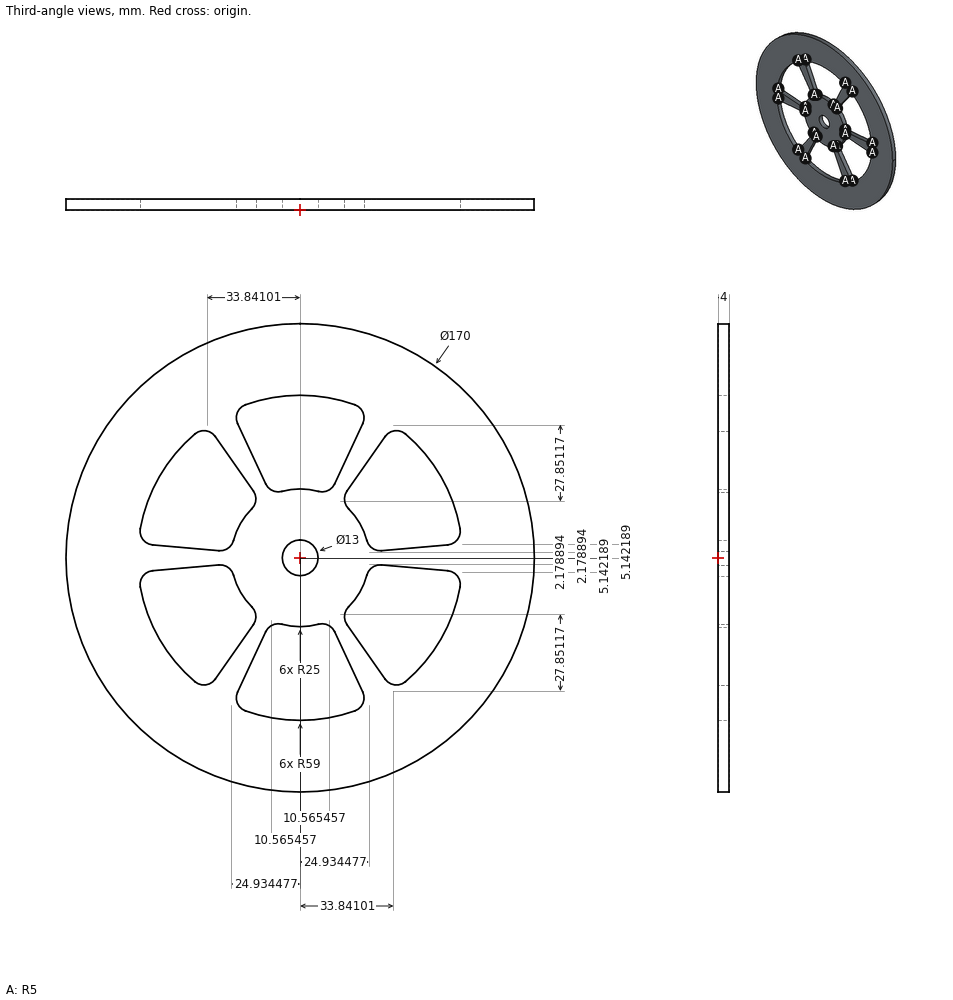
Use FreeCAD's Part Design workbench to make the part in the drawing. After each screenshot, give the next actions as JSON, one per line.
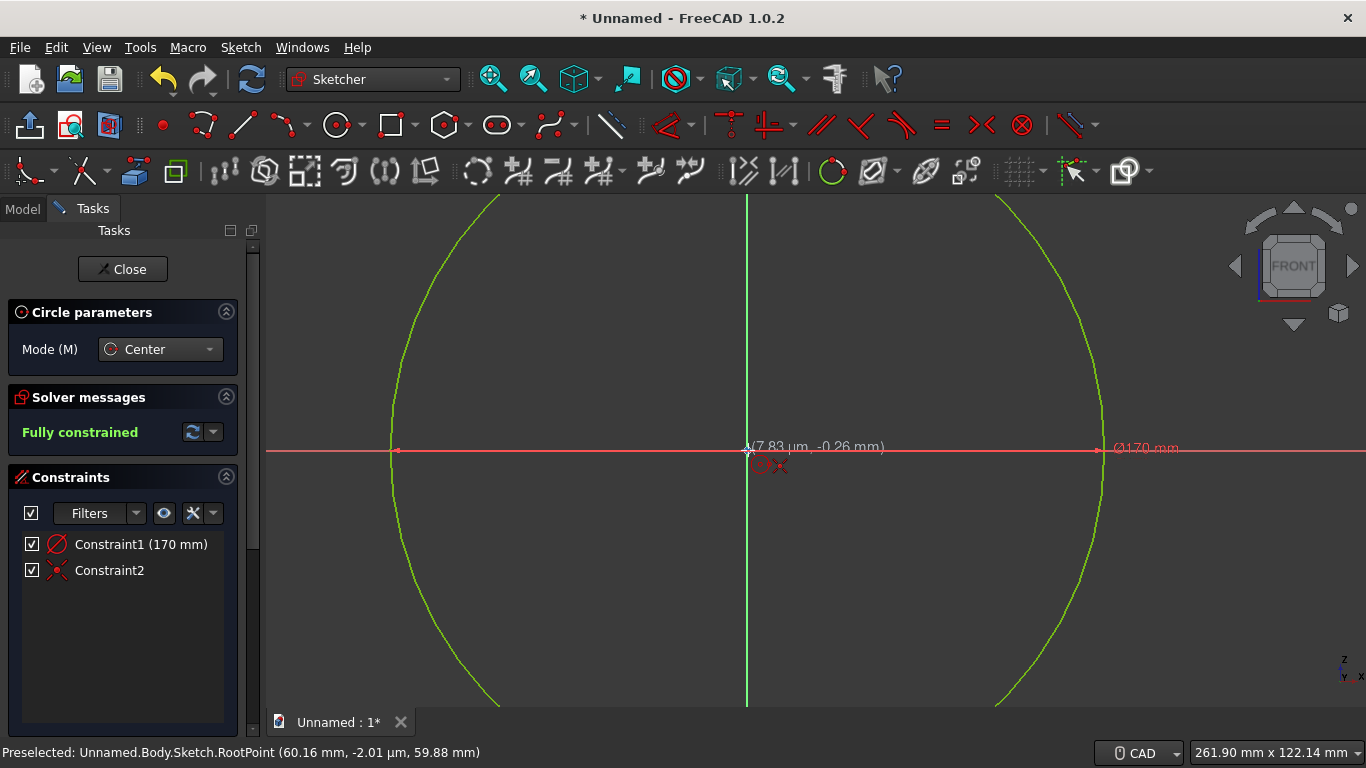
{"action": "left_click", "coordinate": [747, 450]}
{"action": "mouse_move", "coordinate": [767, 431]}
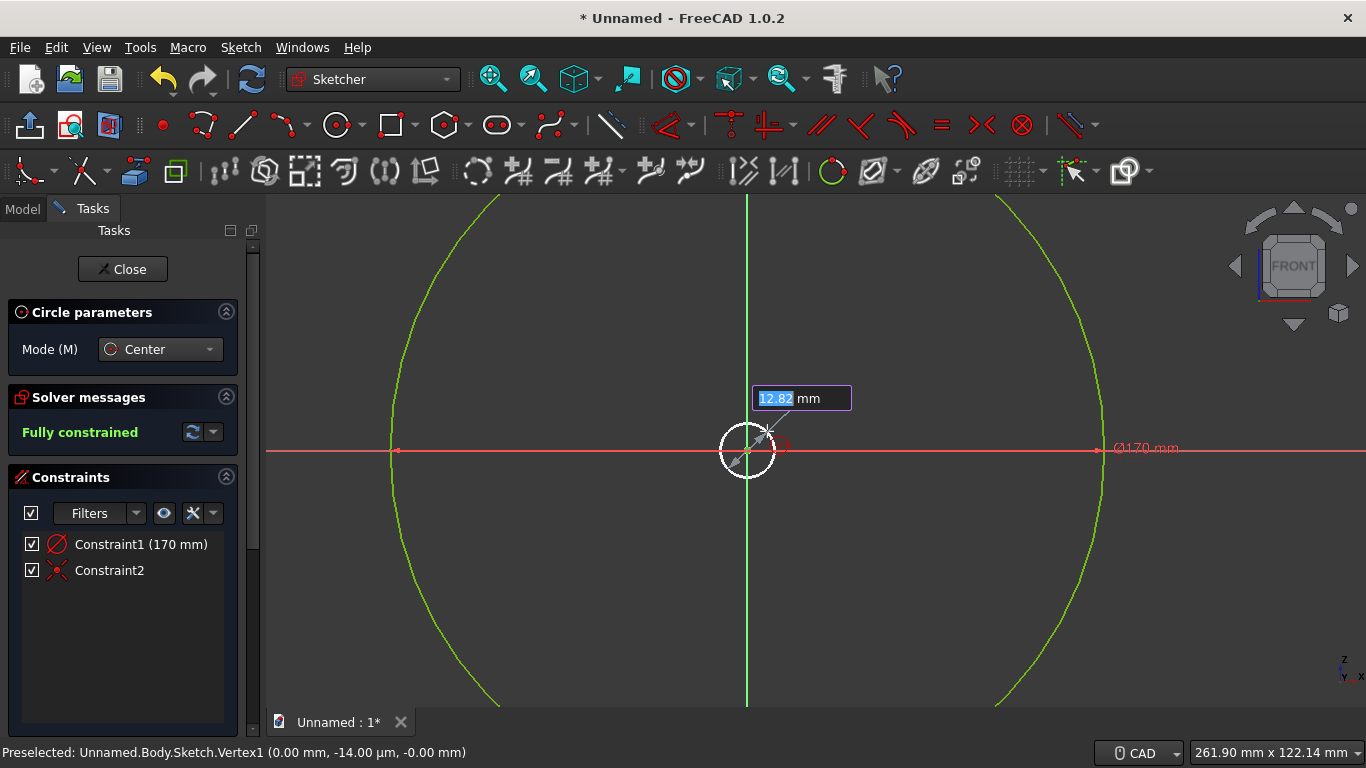
{"action": "type", "text": "13"}
{"action": "key", "text": "Return"}
{"action": "key", "text": "Escape"}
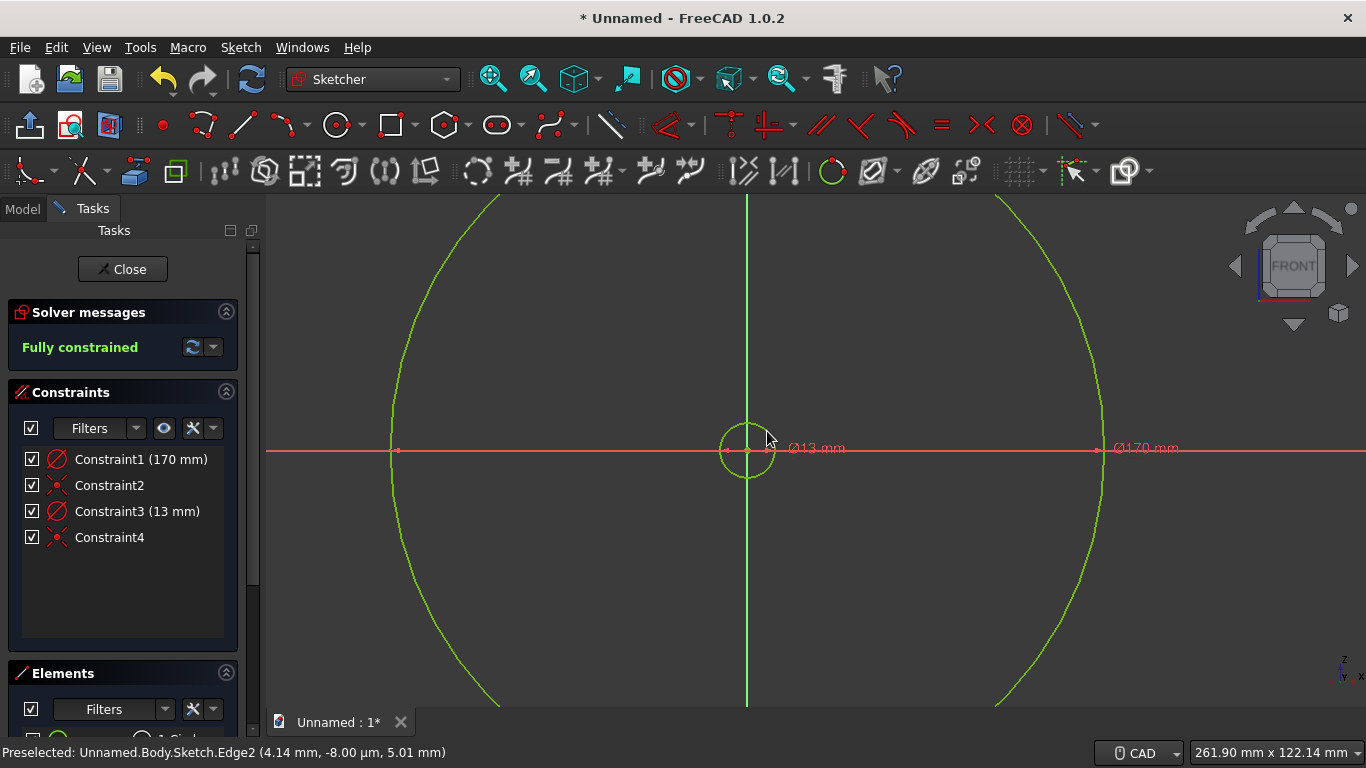
{"action": "left_click", "coordinate": [123, 269]}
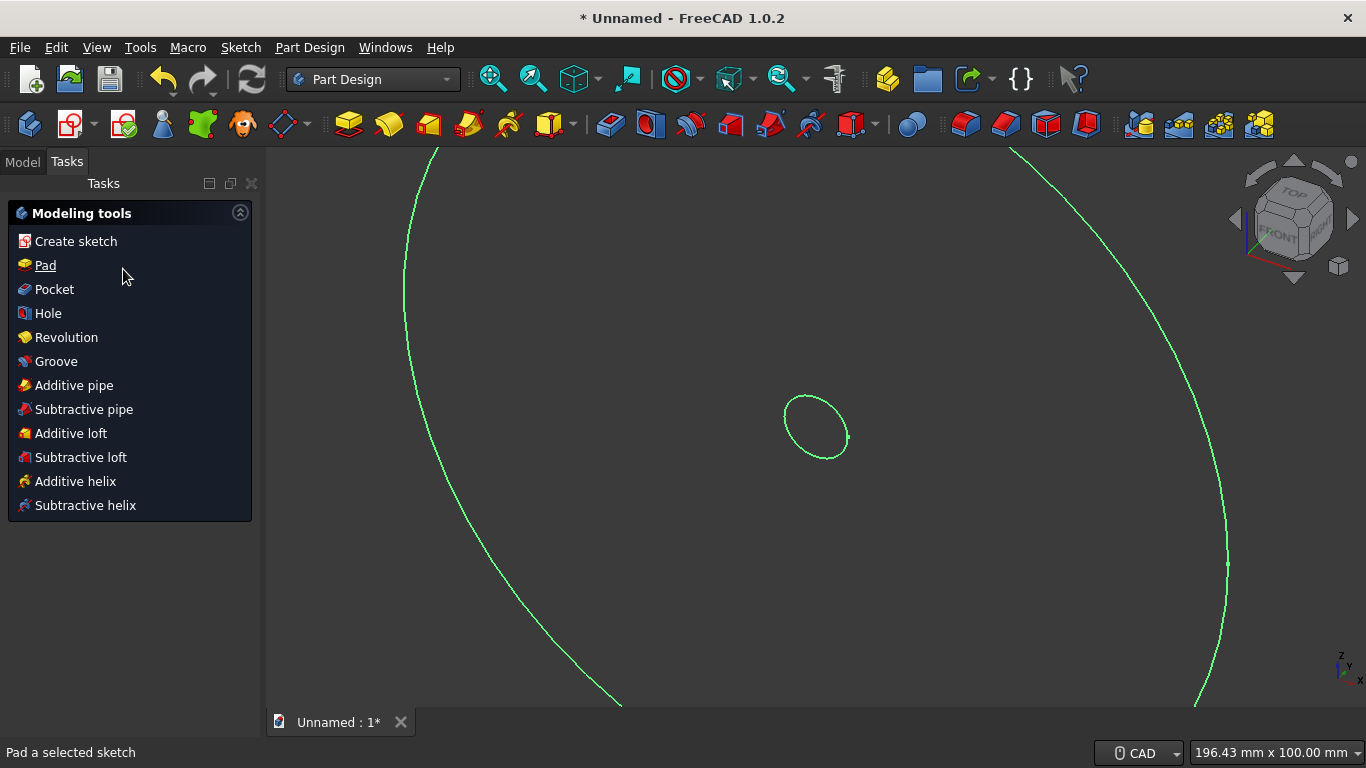
{"action": "left_click", "coordinate": [350, 124]}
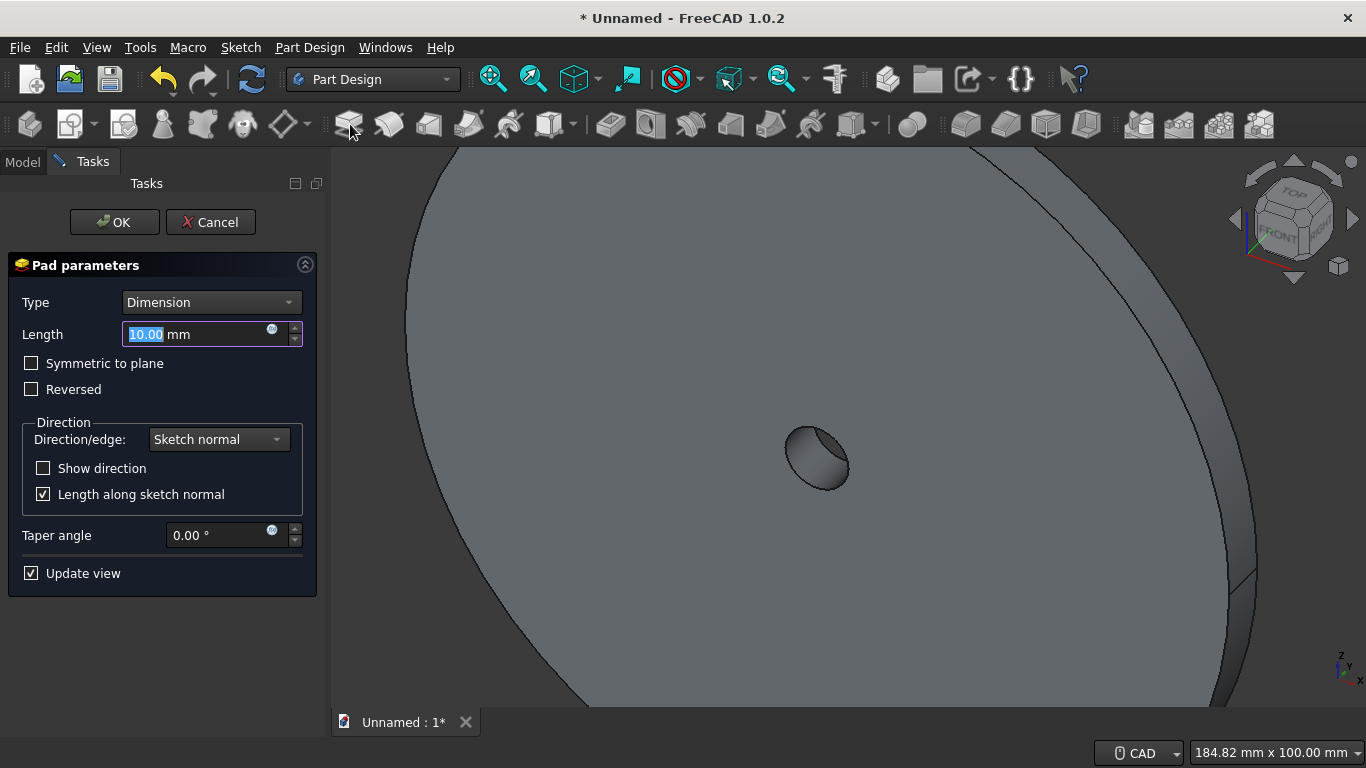
{"action": "type", "text": "4"}
{"action": "key", "text": "Tab"}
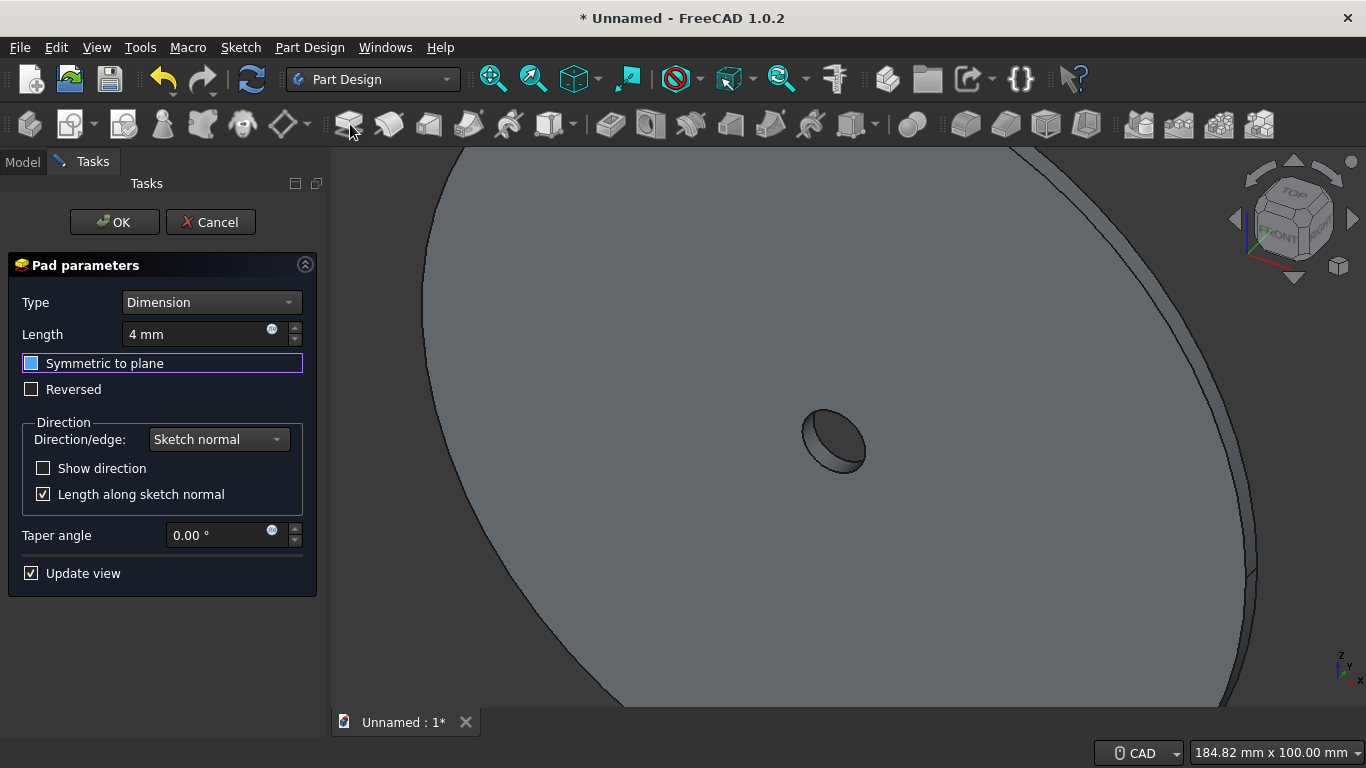
{"action": "left_click", "coordinate": [30, 389]}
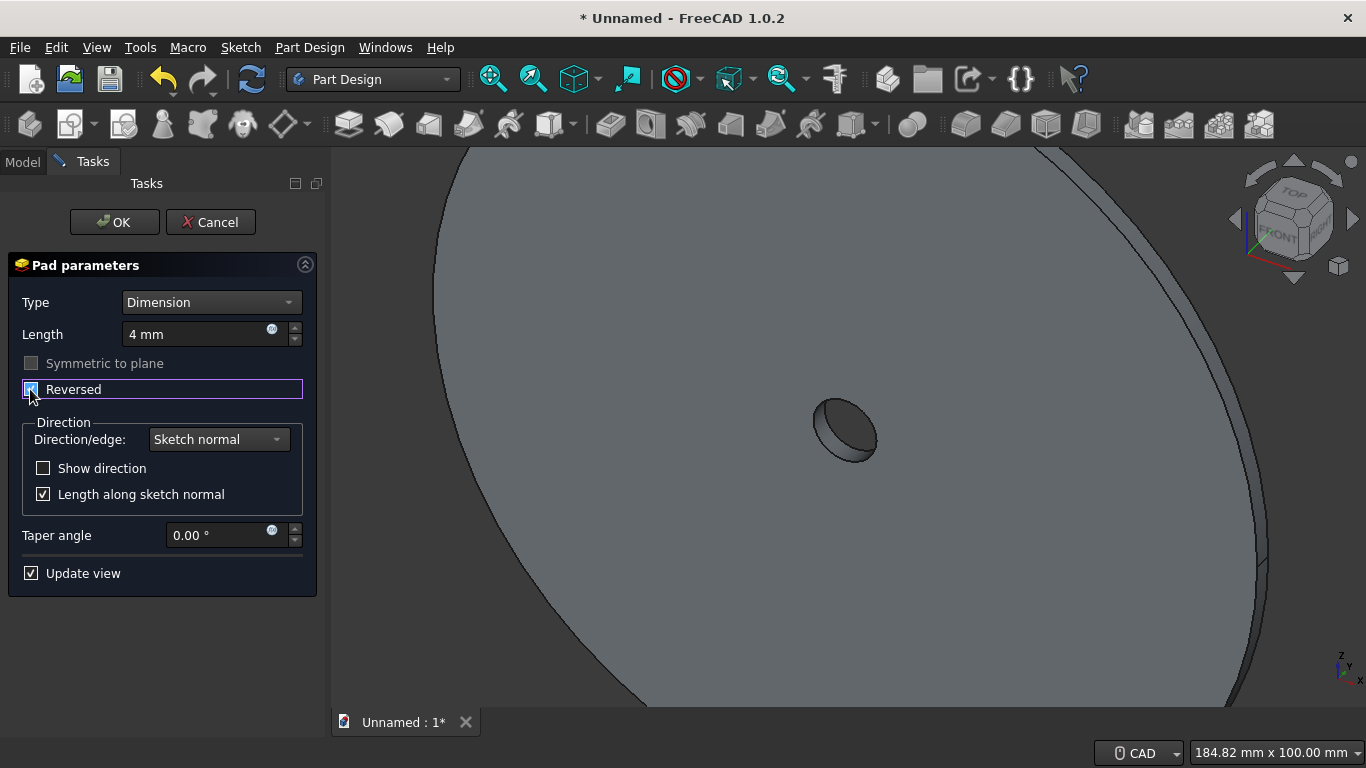
{"action": "left_click", "coordinate": [115, 222]}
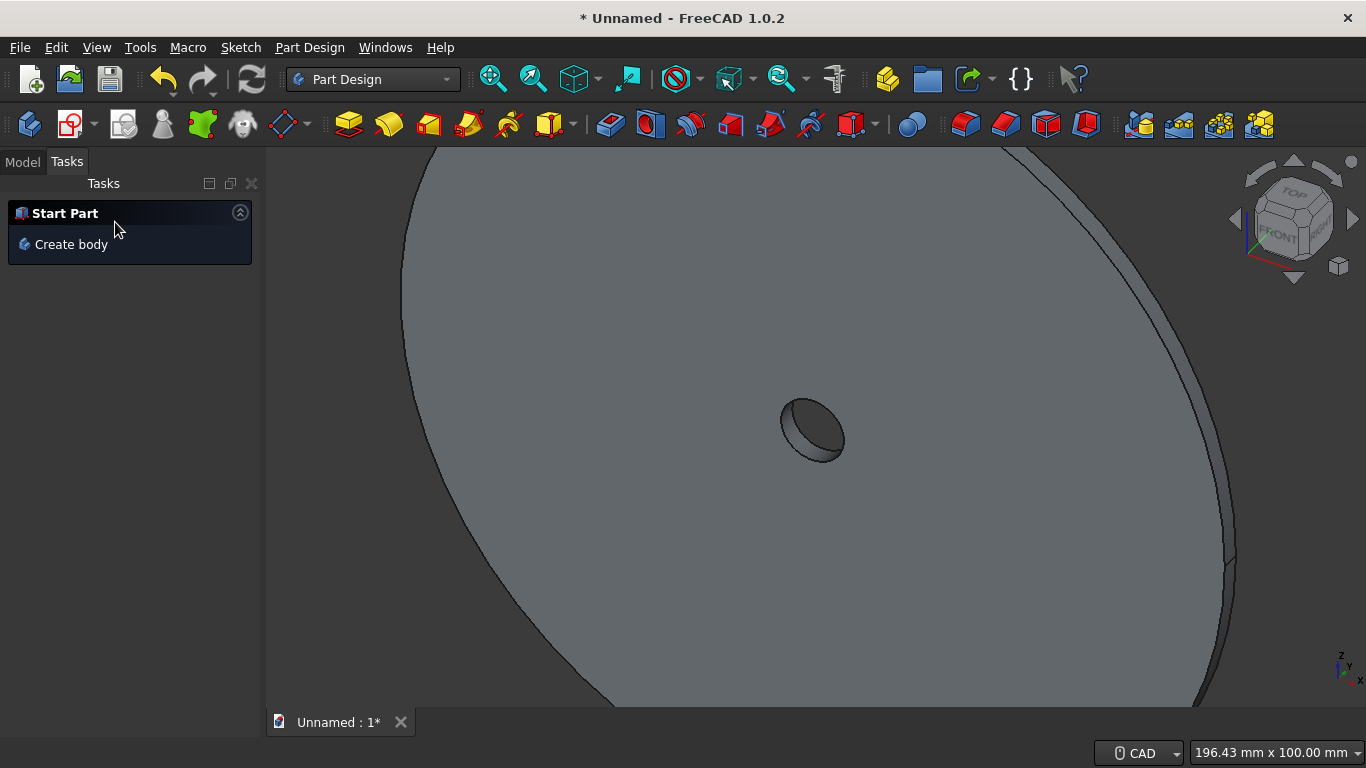
{"action": "left_click", "coordinate": [494, 80]}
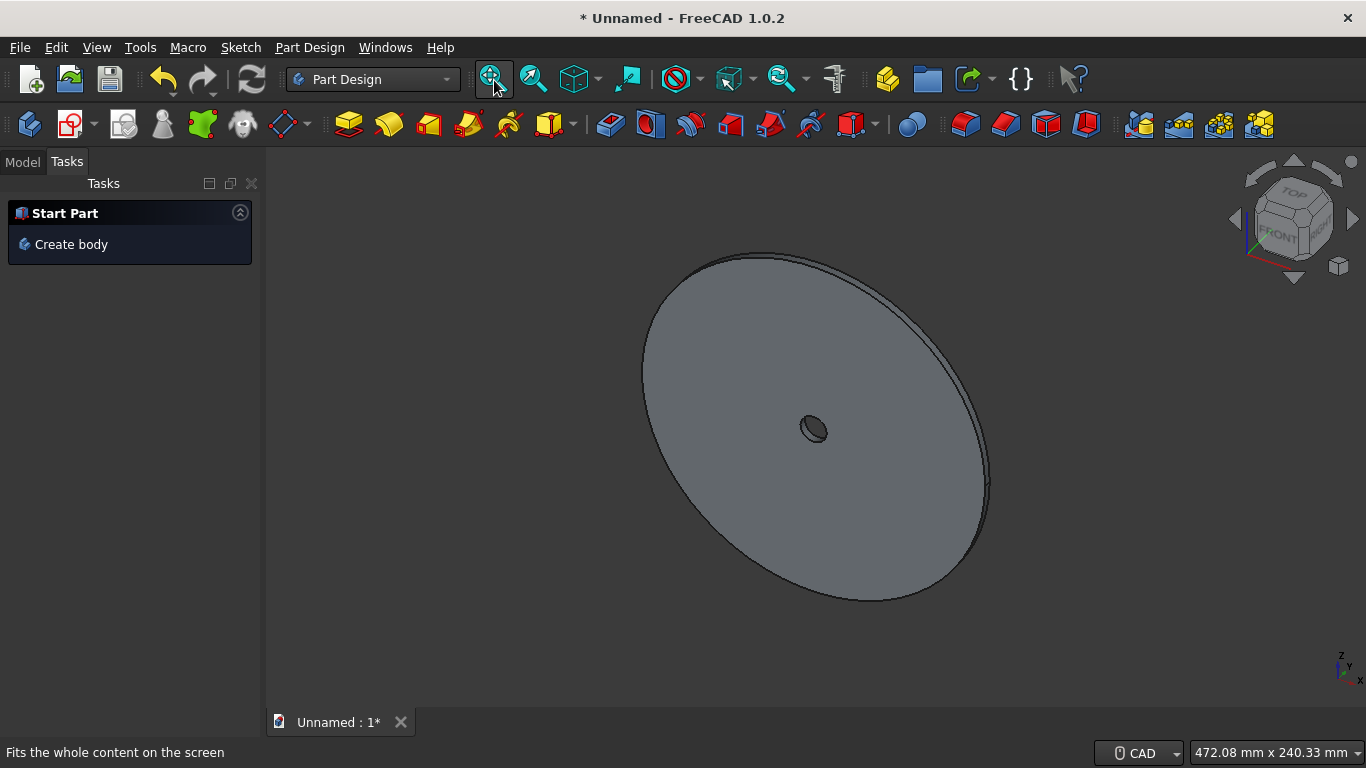
{"action": "key", "text": "4"}